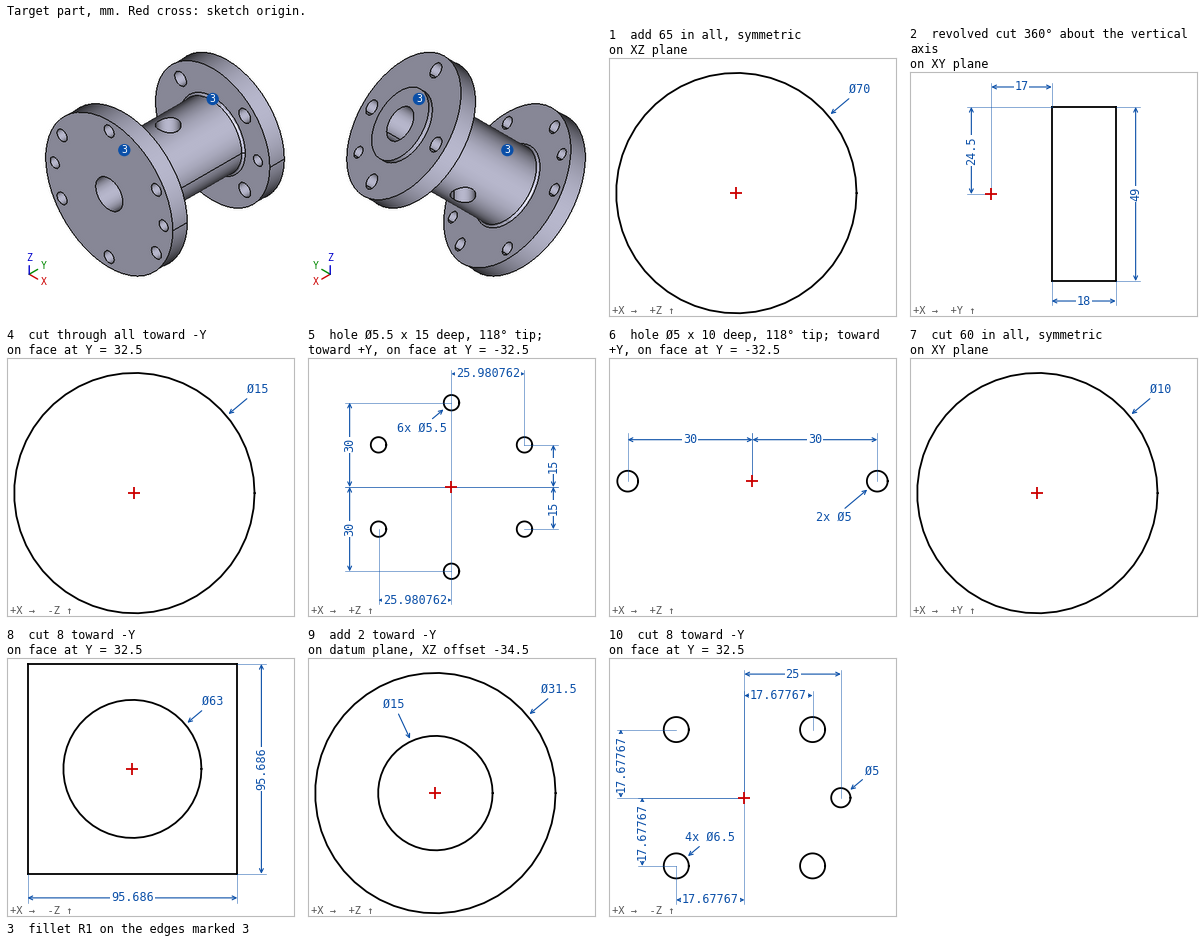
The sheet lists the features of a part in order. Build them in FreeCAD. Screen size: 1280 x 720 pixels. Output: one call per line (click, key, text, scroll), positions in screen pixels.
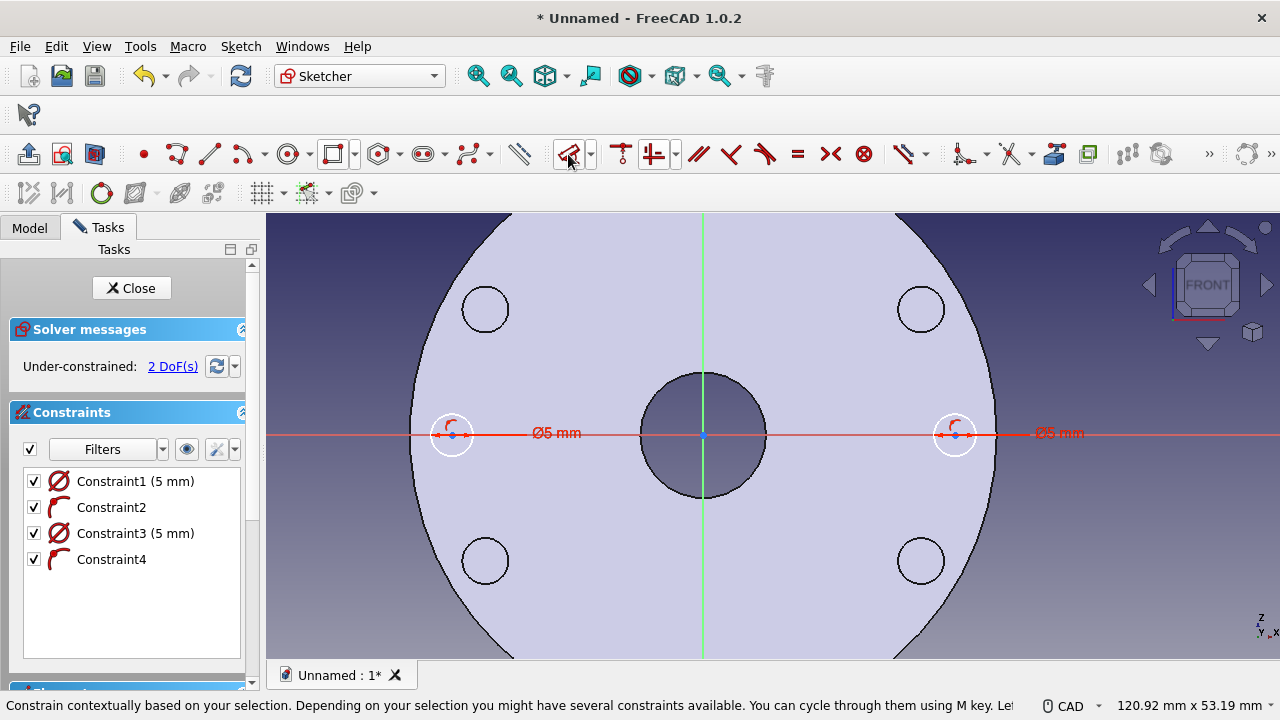
click(955, 435)
click(829, 469)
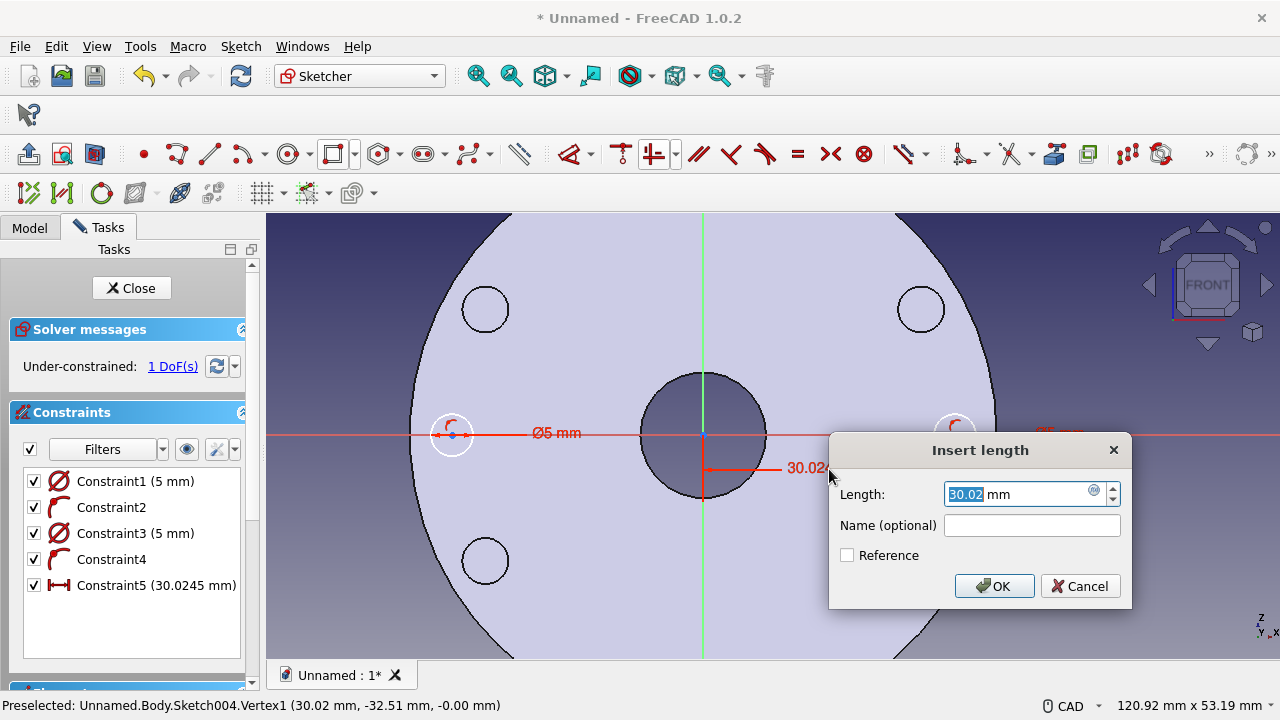
text(30)
key(Return)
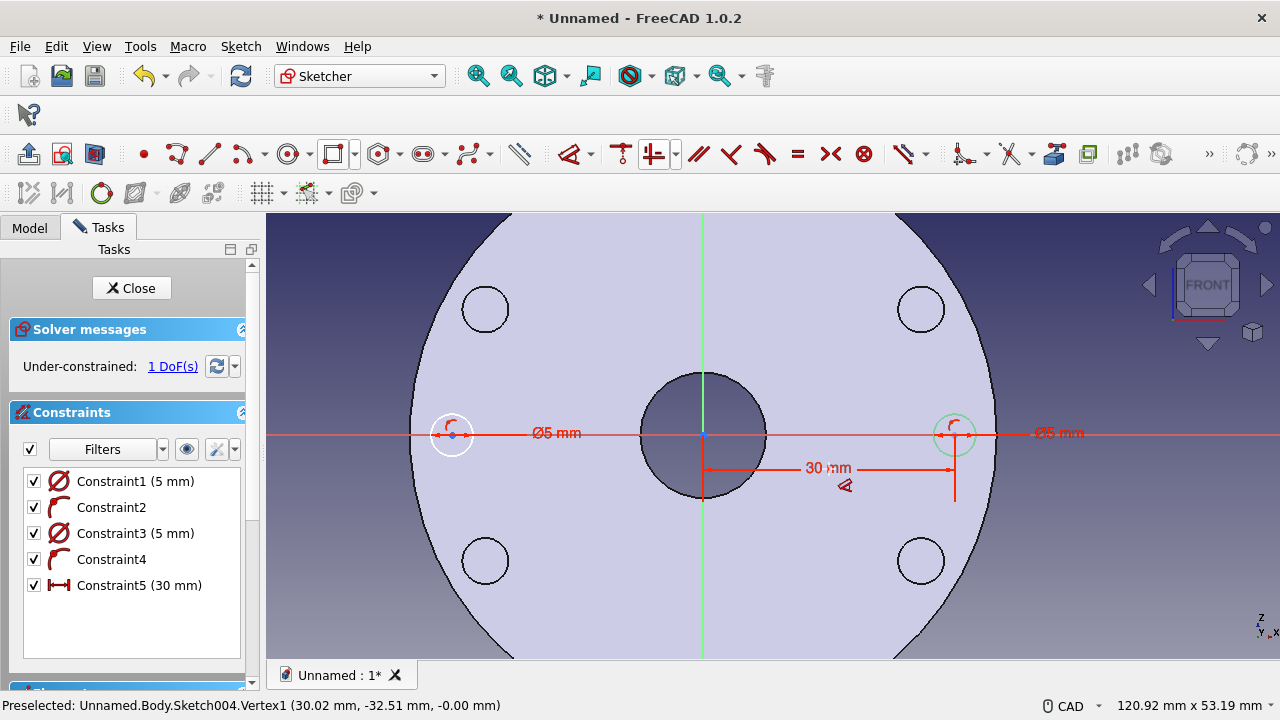
click(452, 435)
click(578, 469)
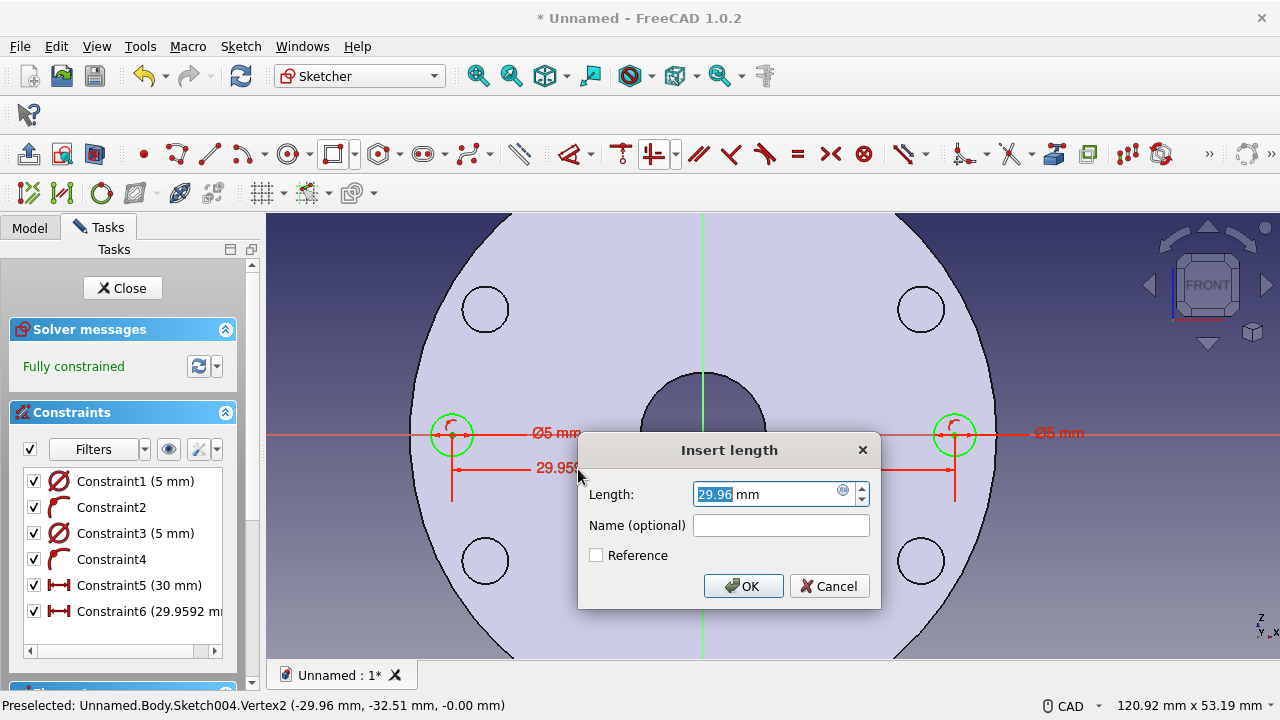
text(30)
key(Return)
key(Escape)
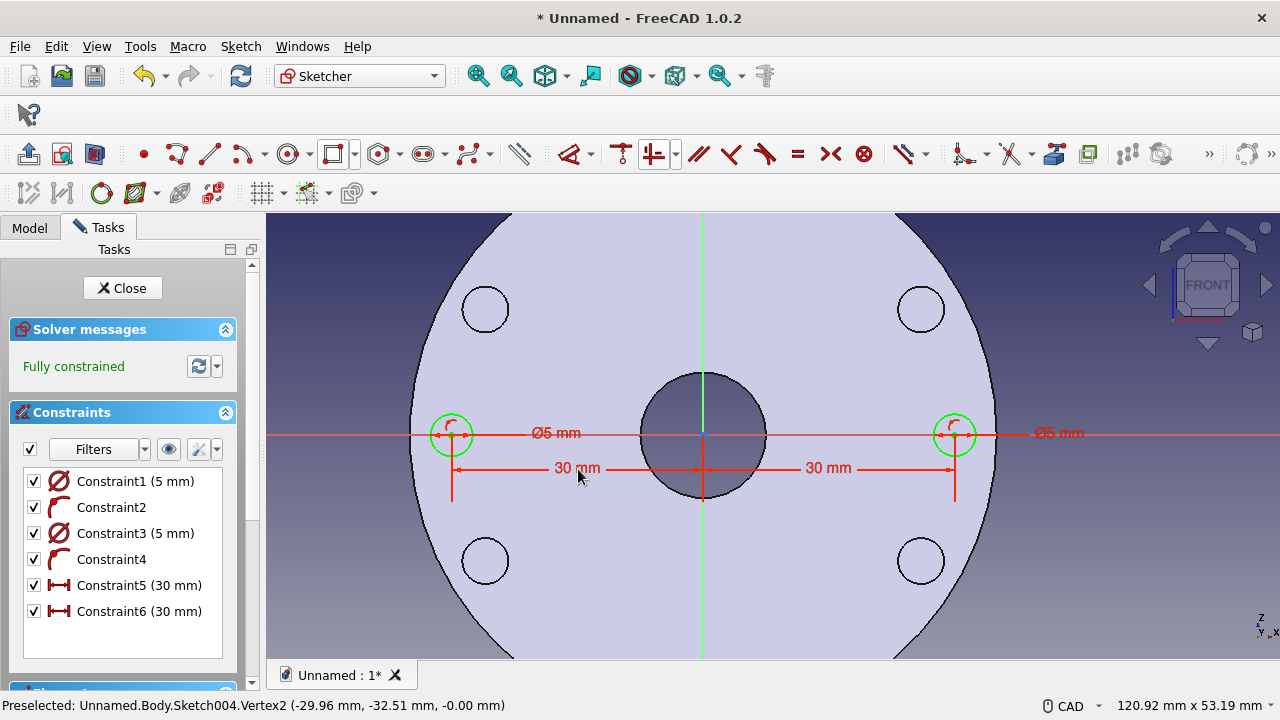
click(123, 288)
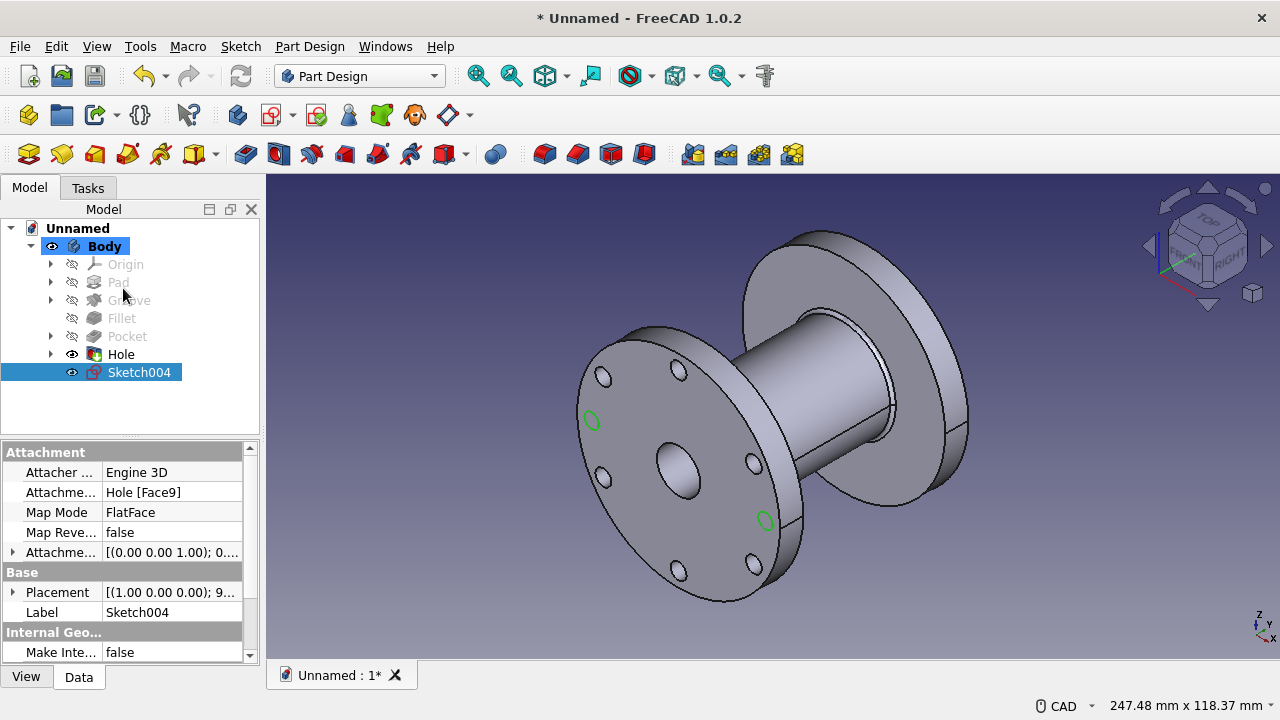
click(279, 154)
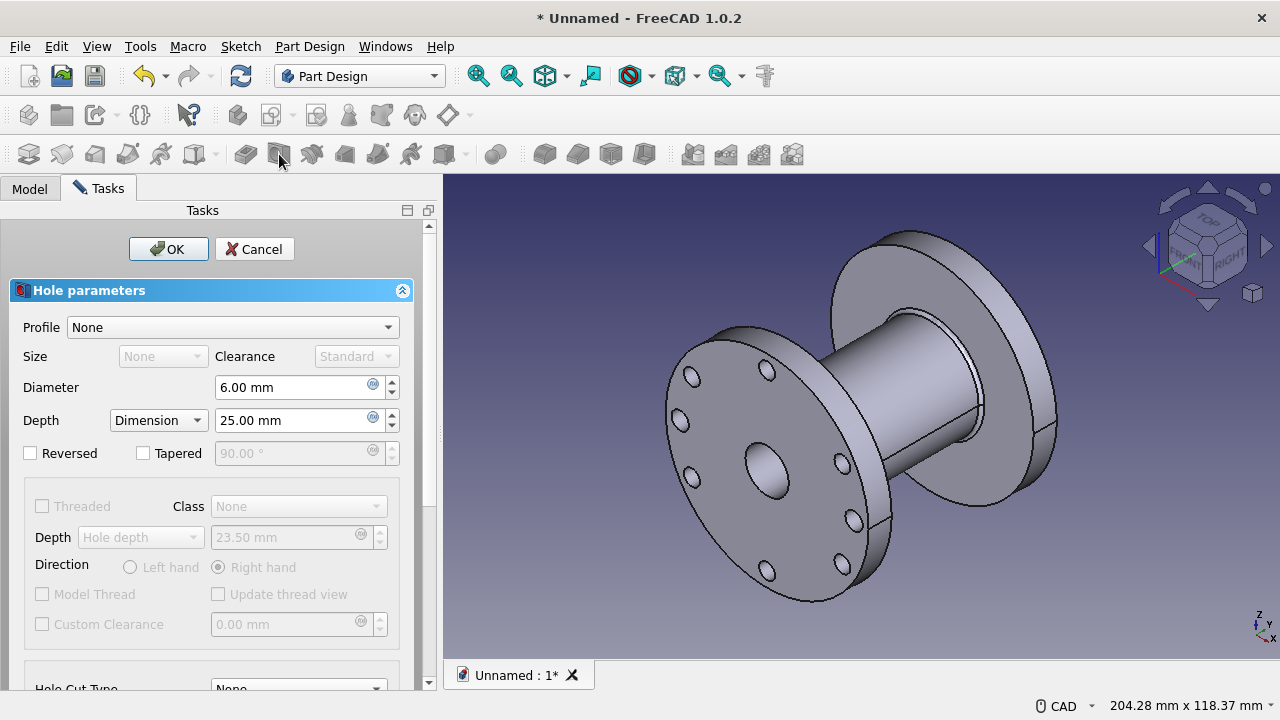
triple_click(300, 388)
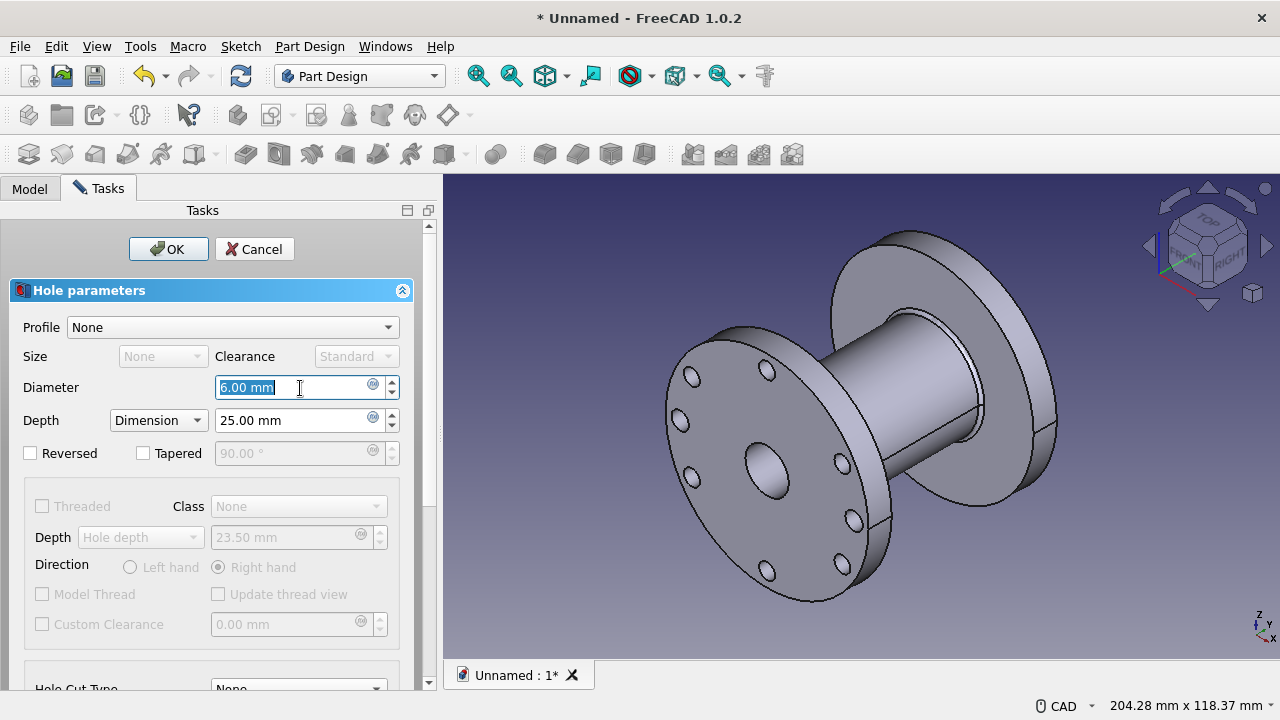
text(5)
key(Tab)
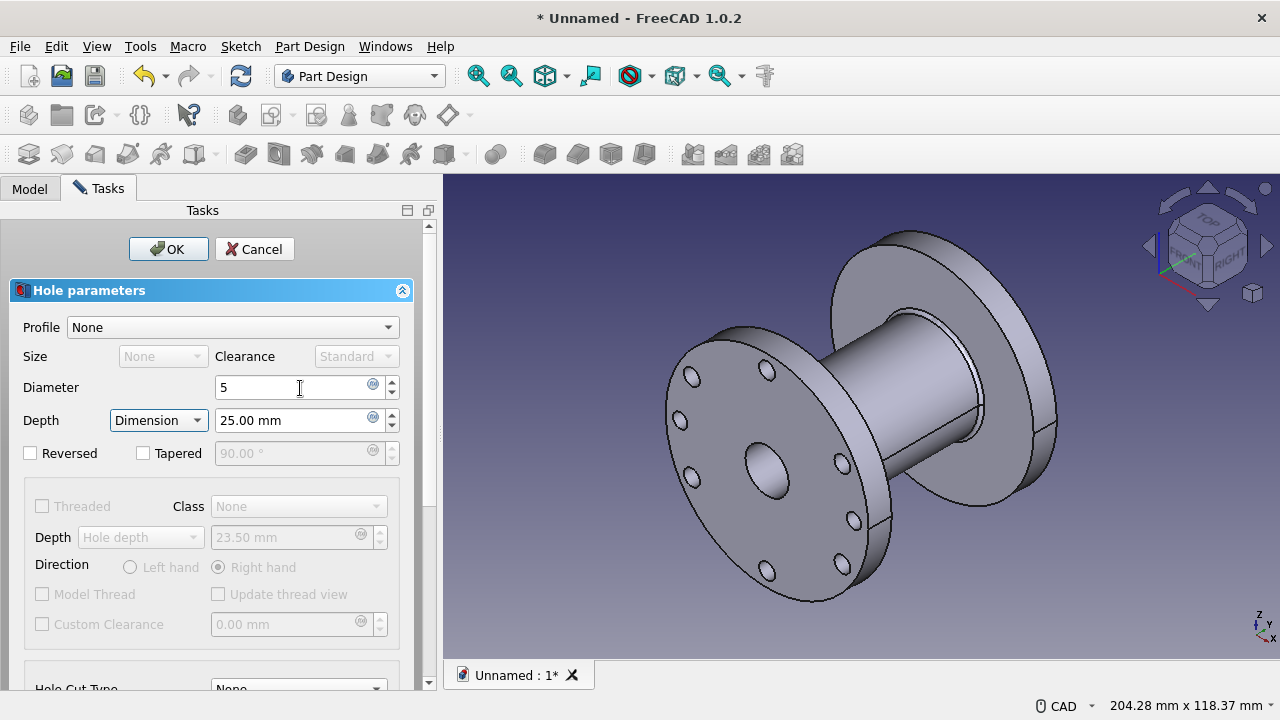
triple_click(300, 420)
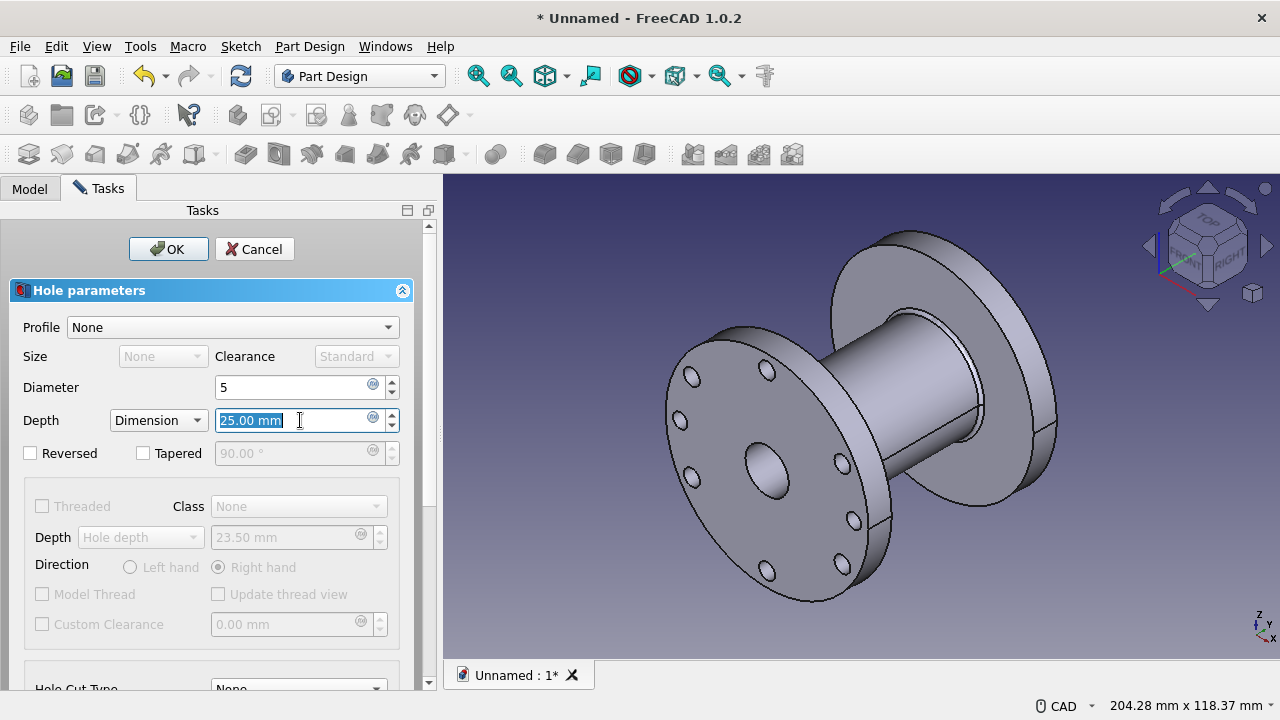
text(10)
key(Tab)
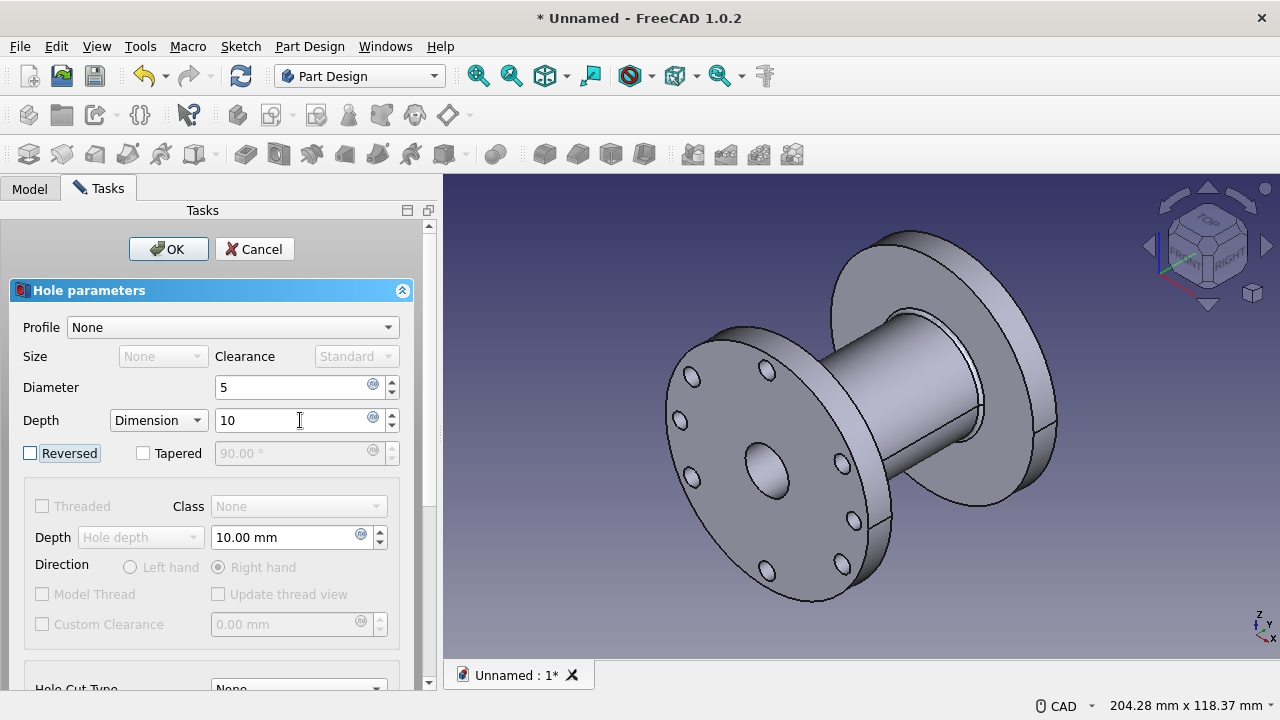
click(169, 249)